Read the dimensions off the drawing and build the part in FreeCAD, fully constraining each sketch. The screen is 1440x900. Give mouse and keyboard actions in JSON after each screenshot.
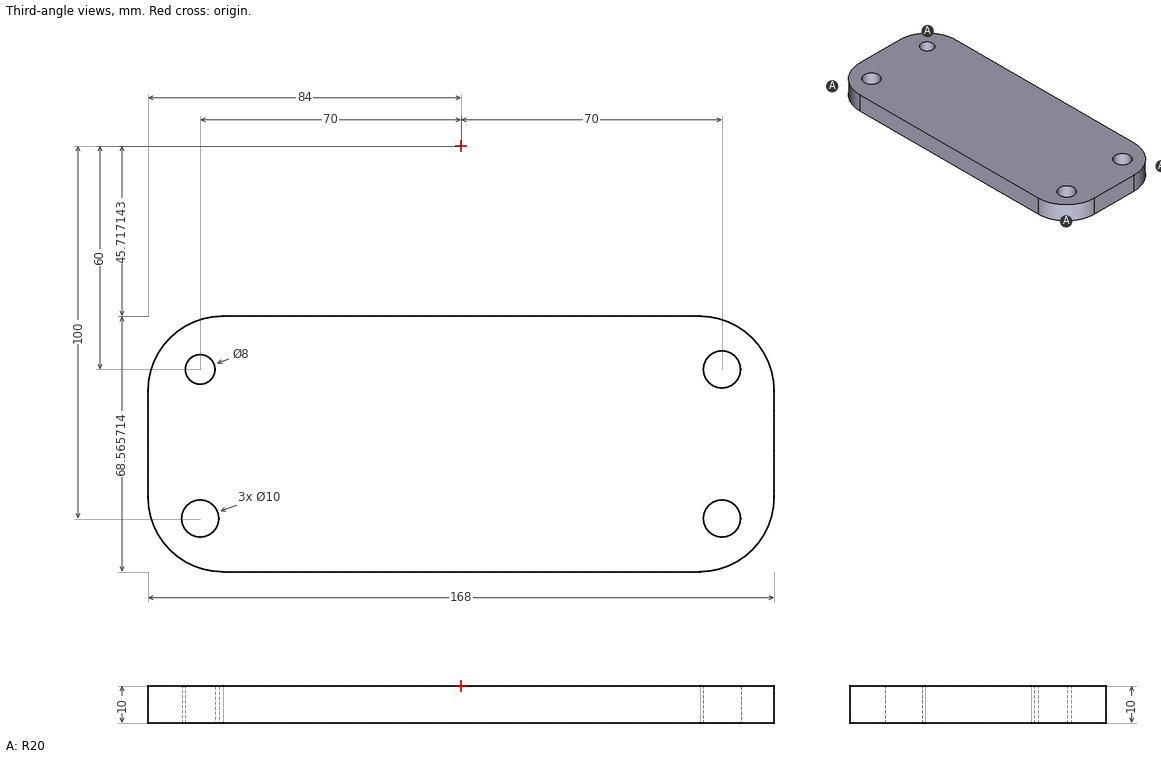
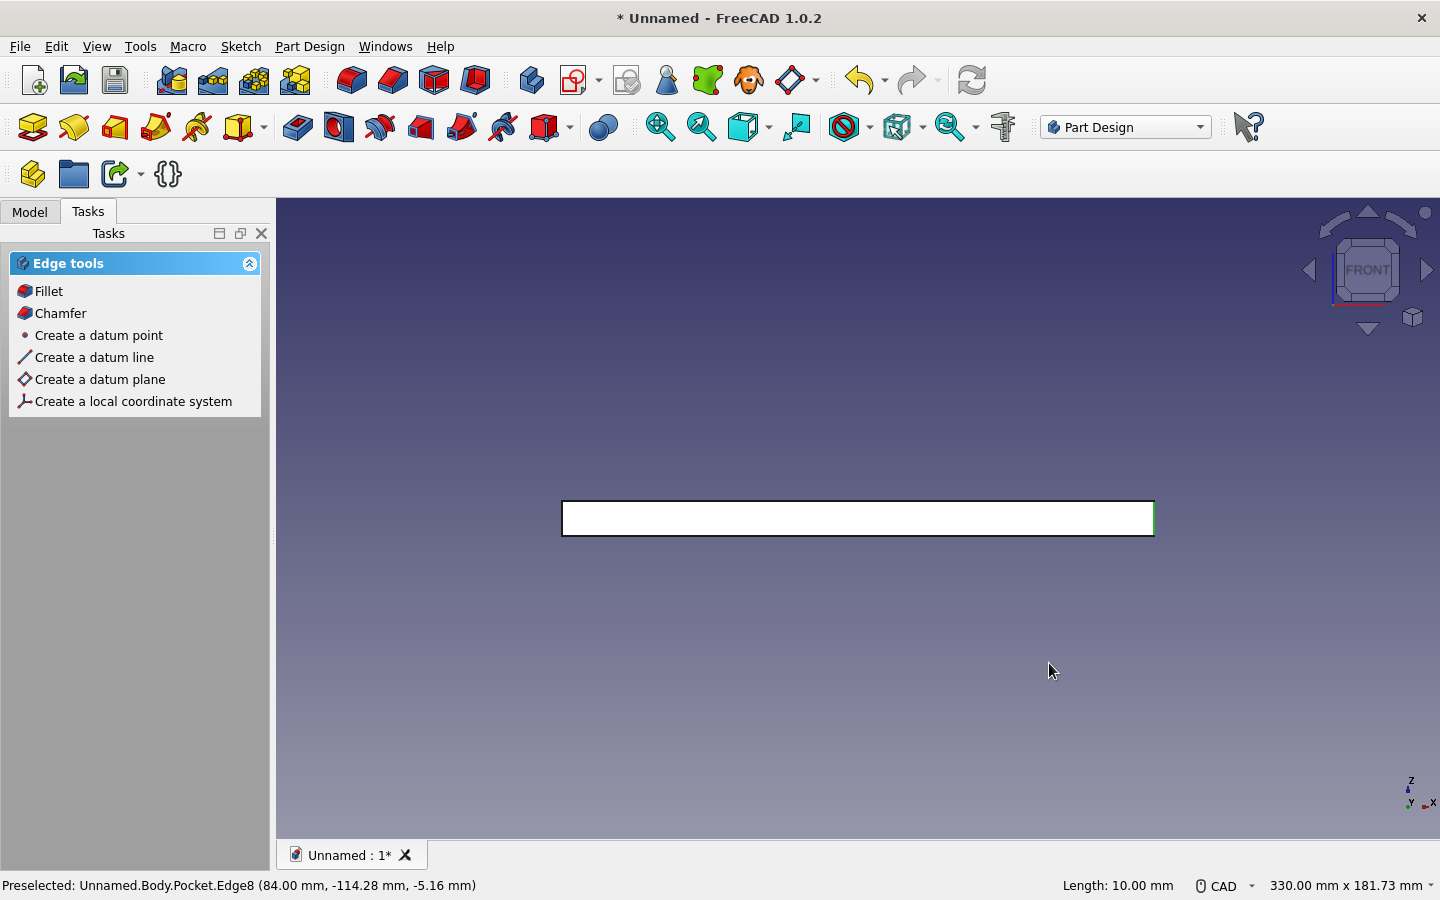
{"action": "left_click", "coordinate": [562, 517], "text": "ctrl"}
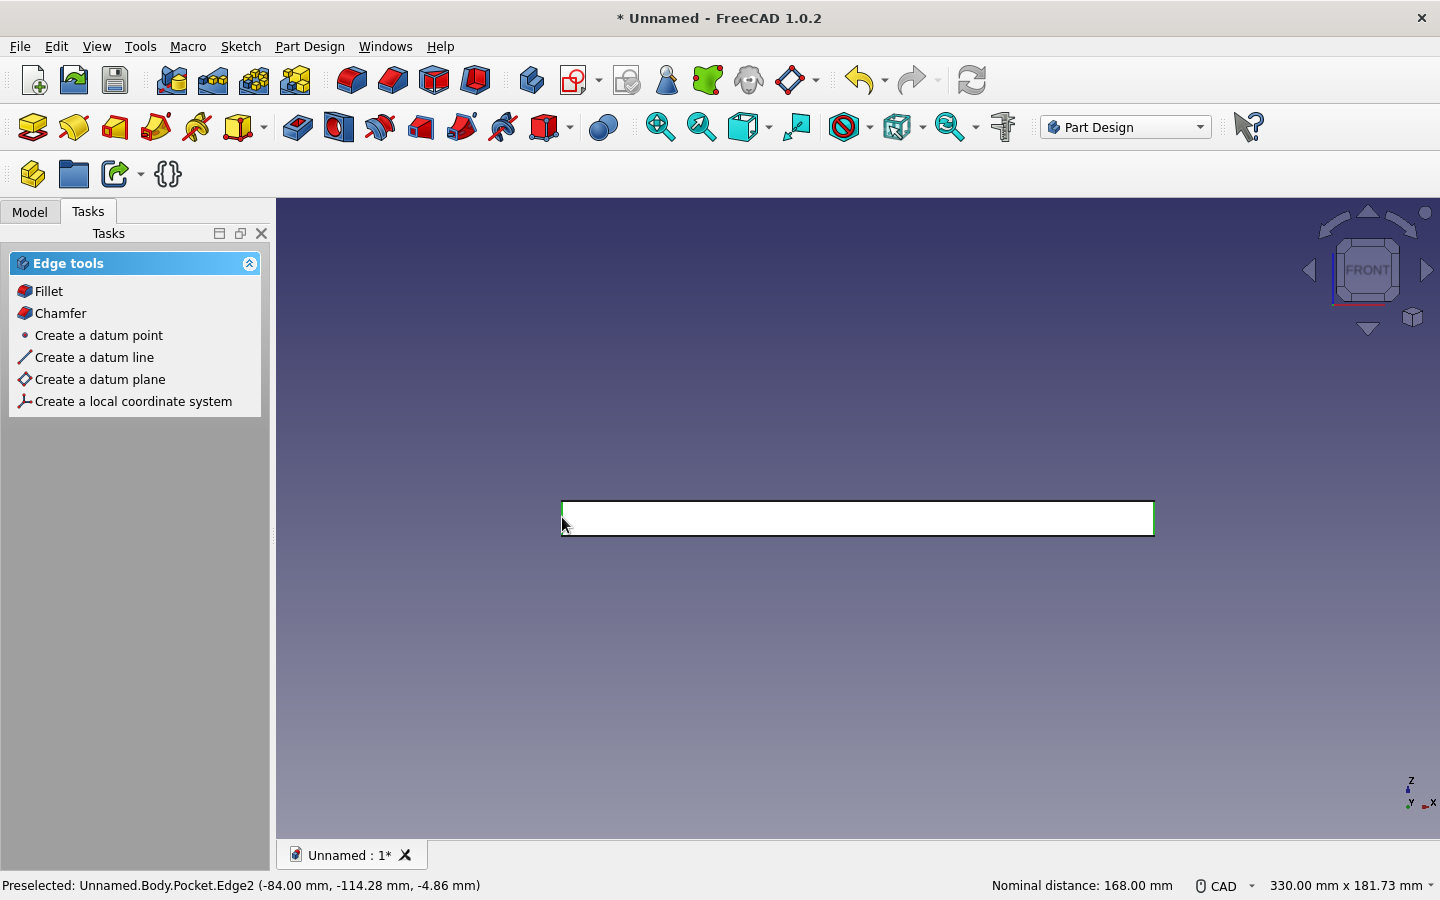
{"action": "key", "text": "3"}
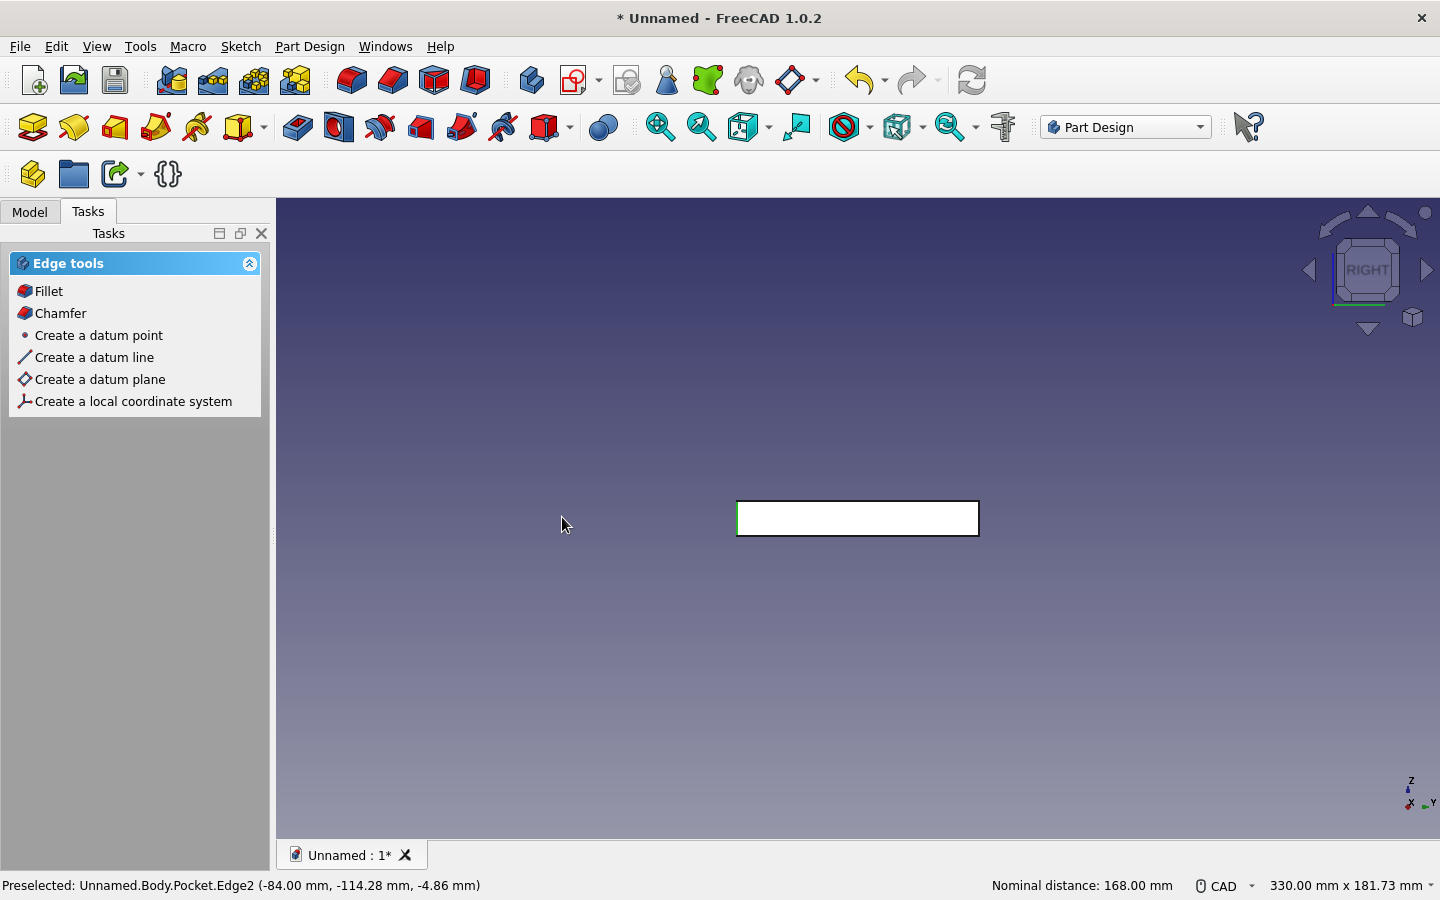
{"action": "left_click", "coordinate": [661, 128]}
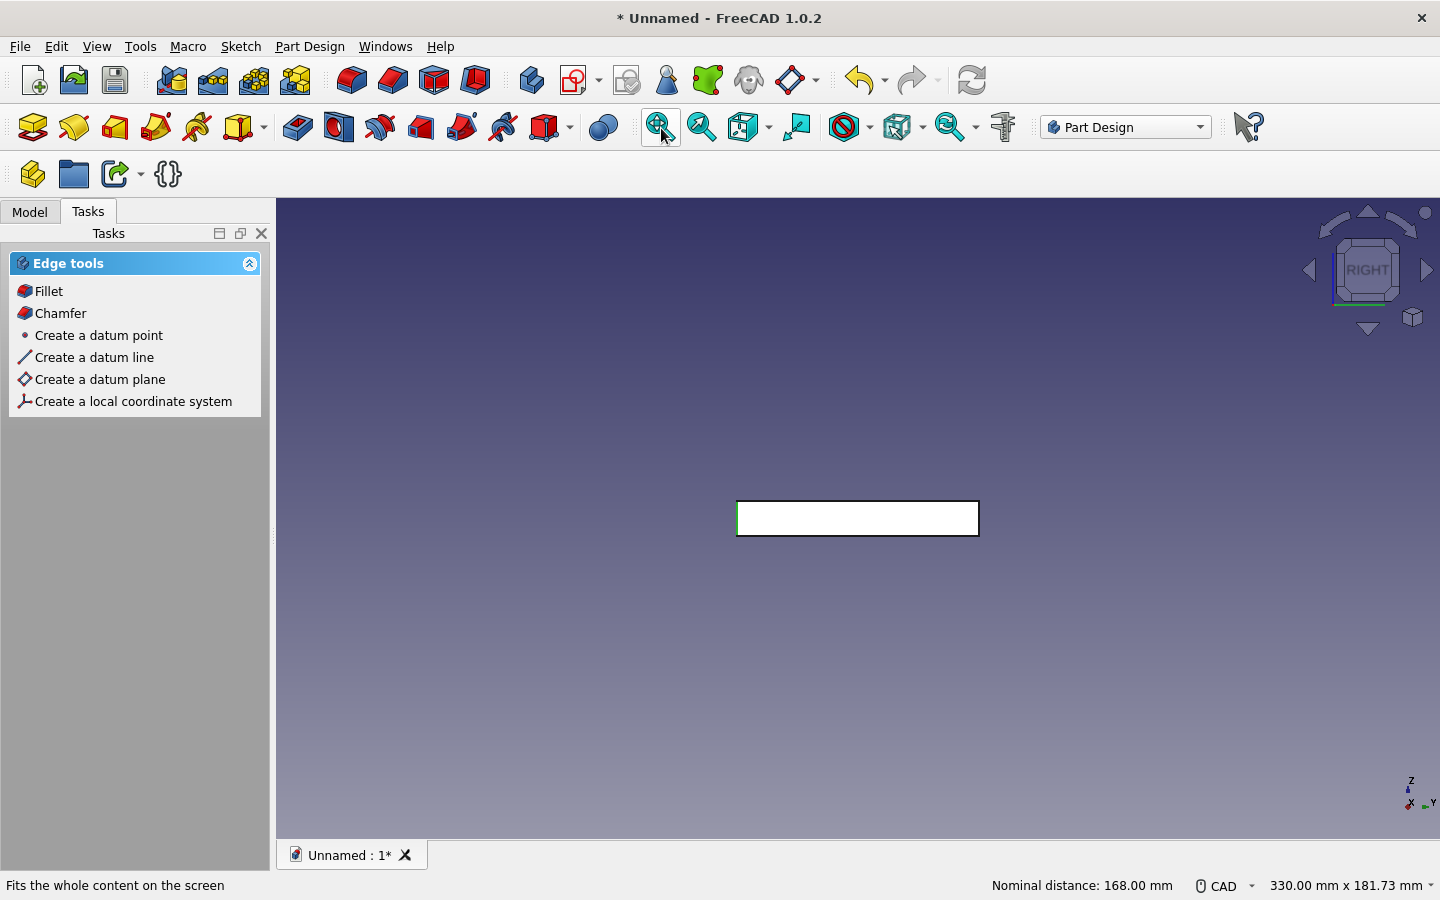
{"action": "left_click", "coordinate": [979, 517], "text": "ctrl"}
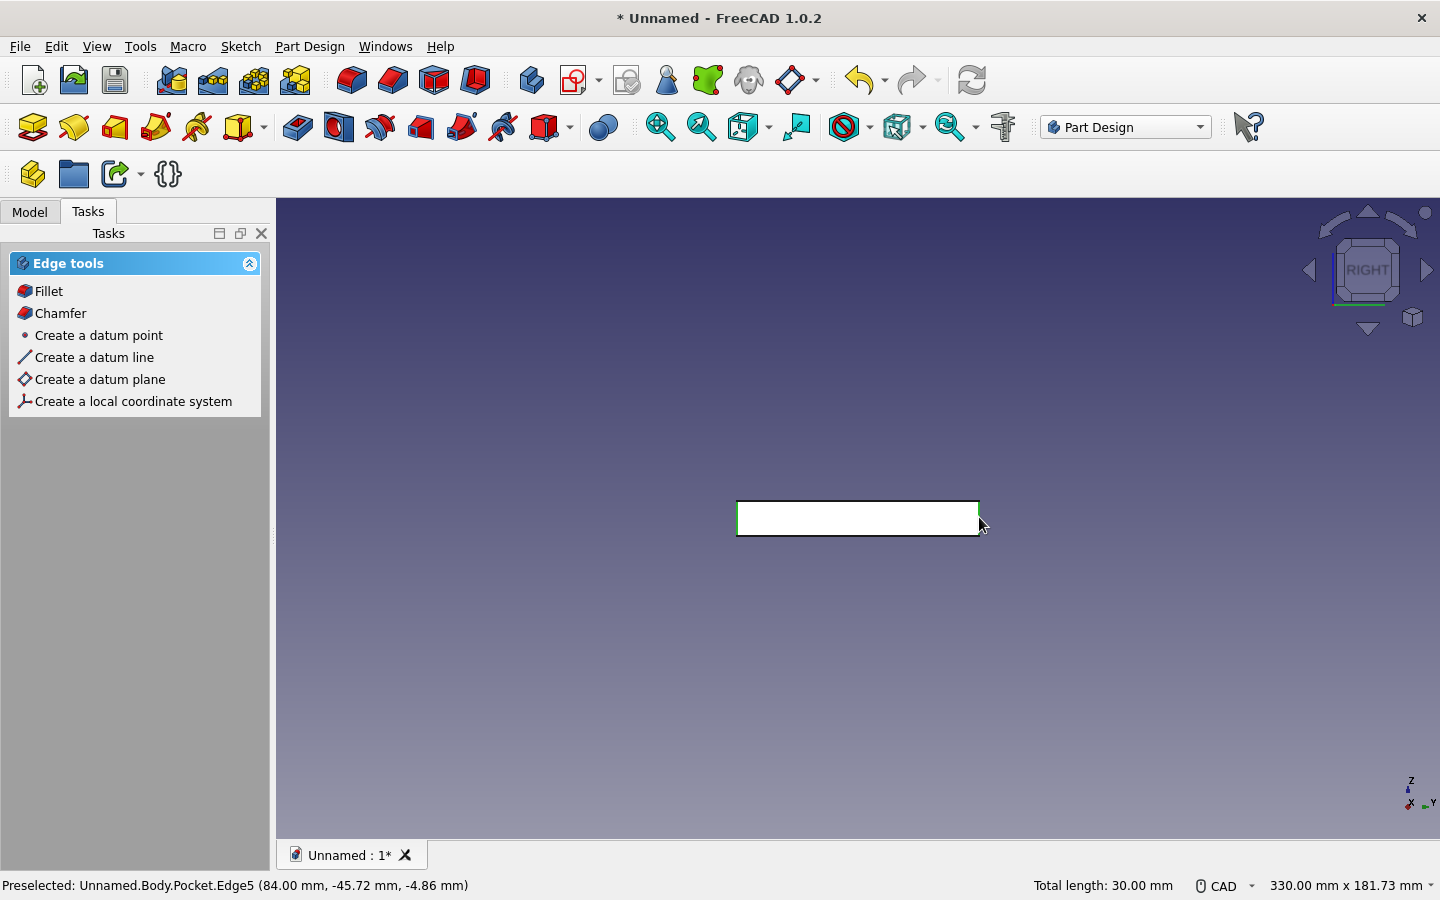
{"action": "key", "text": "5"}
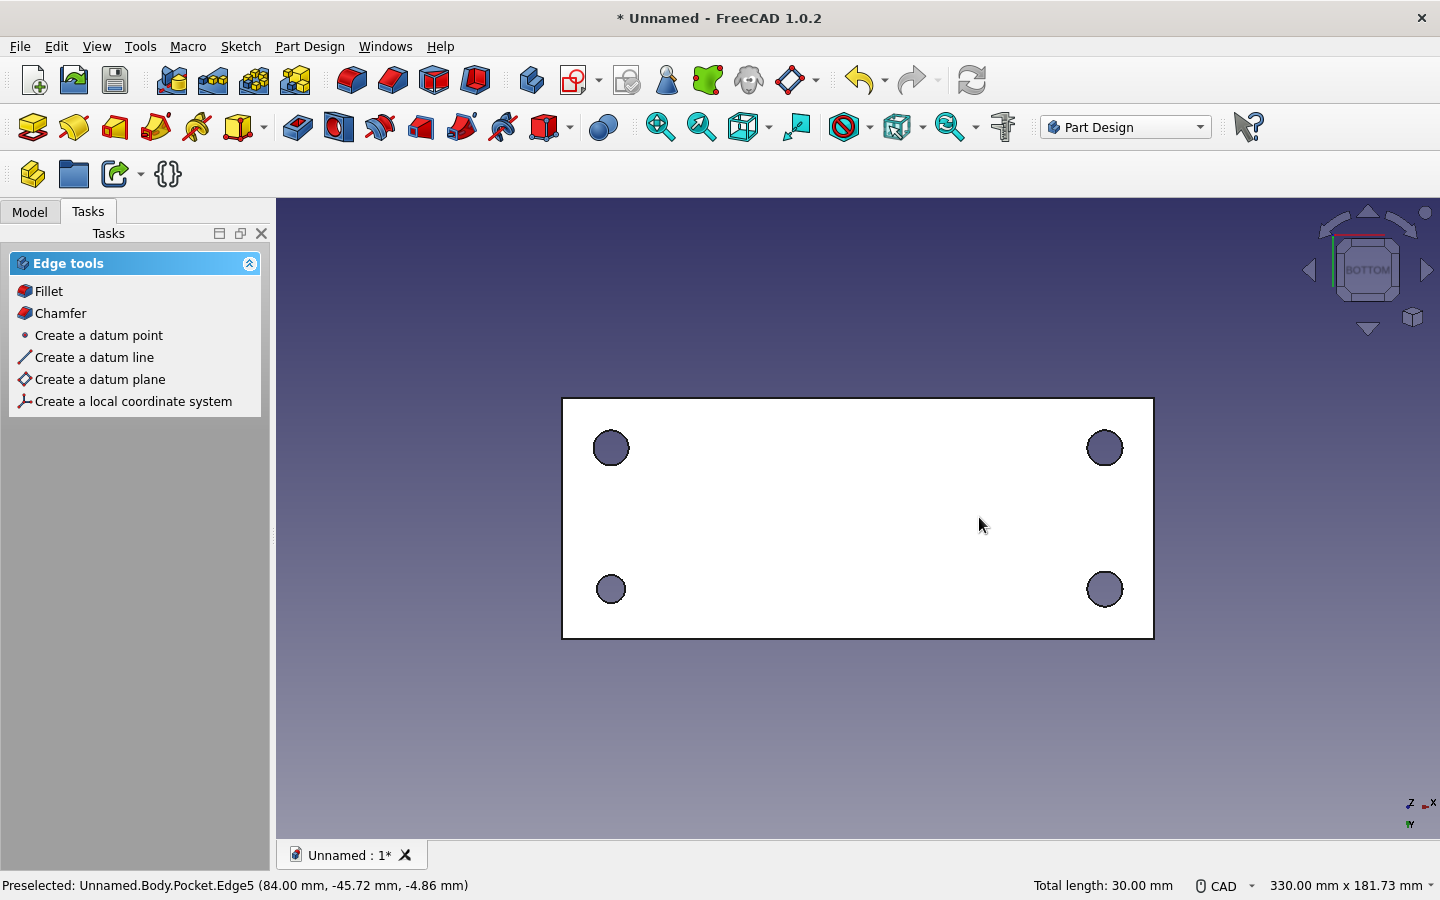
{"action": "key", "text": "4"}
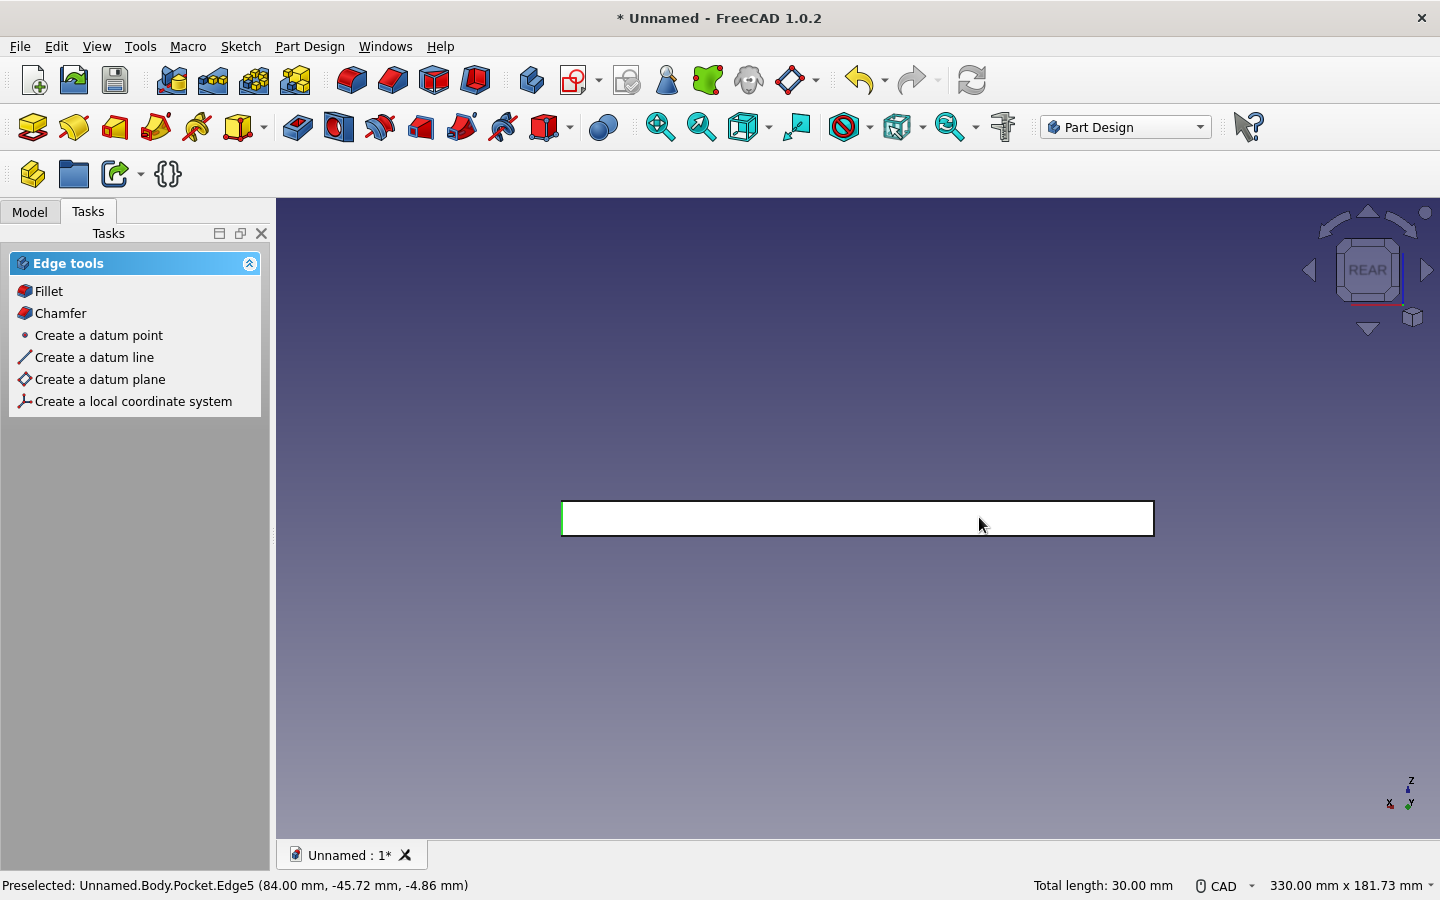
{"action": "left_click", "coordinate": [1154, 517], "text": "ctrl"}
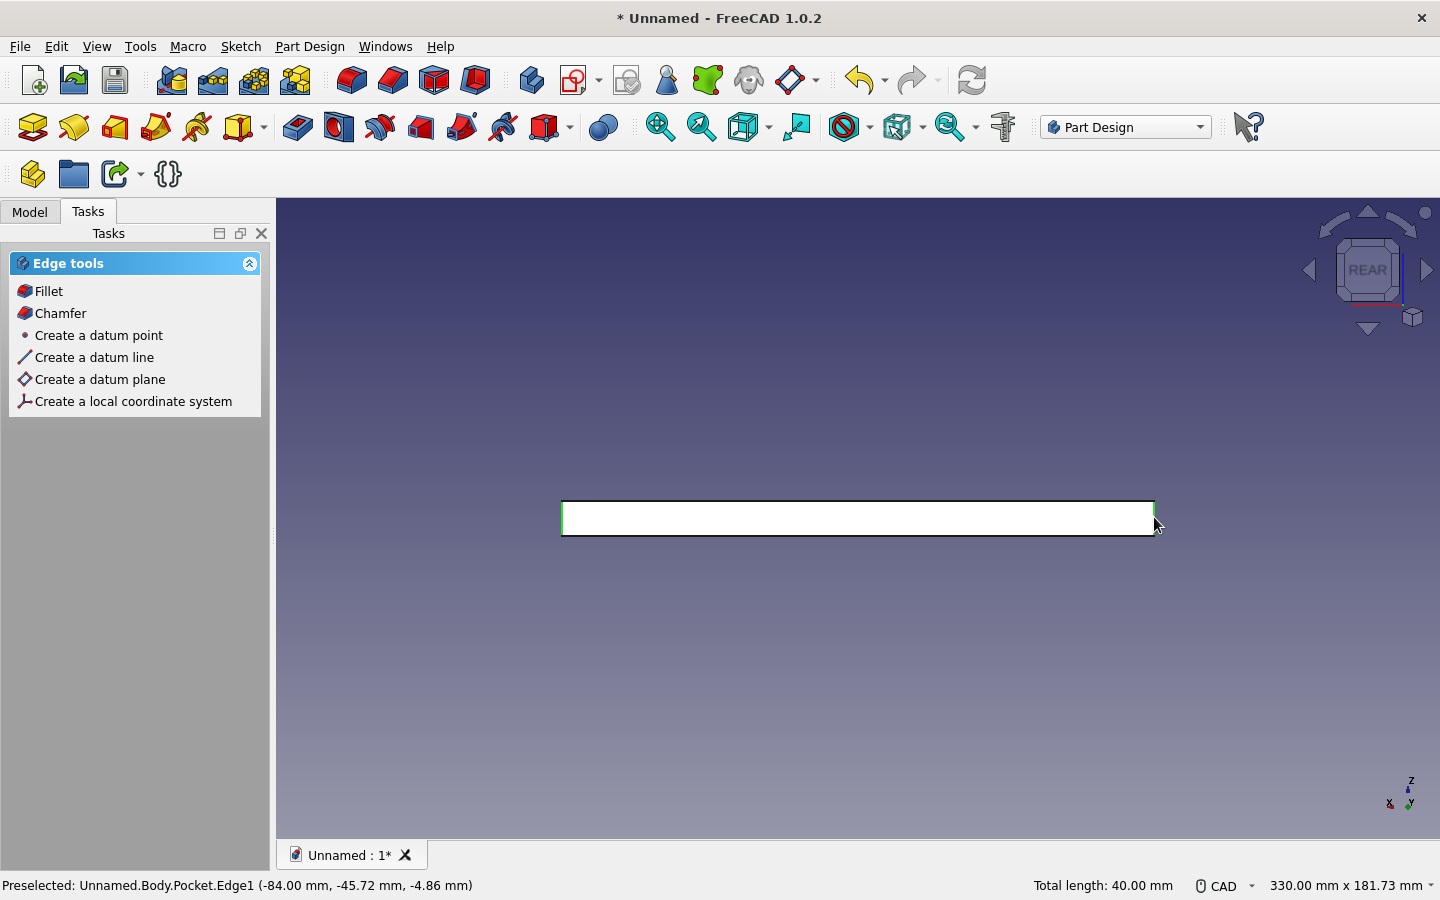
{"action": "left_click", "coordinate": [352, 80]}